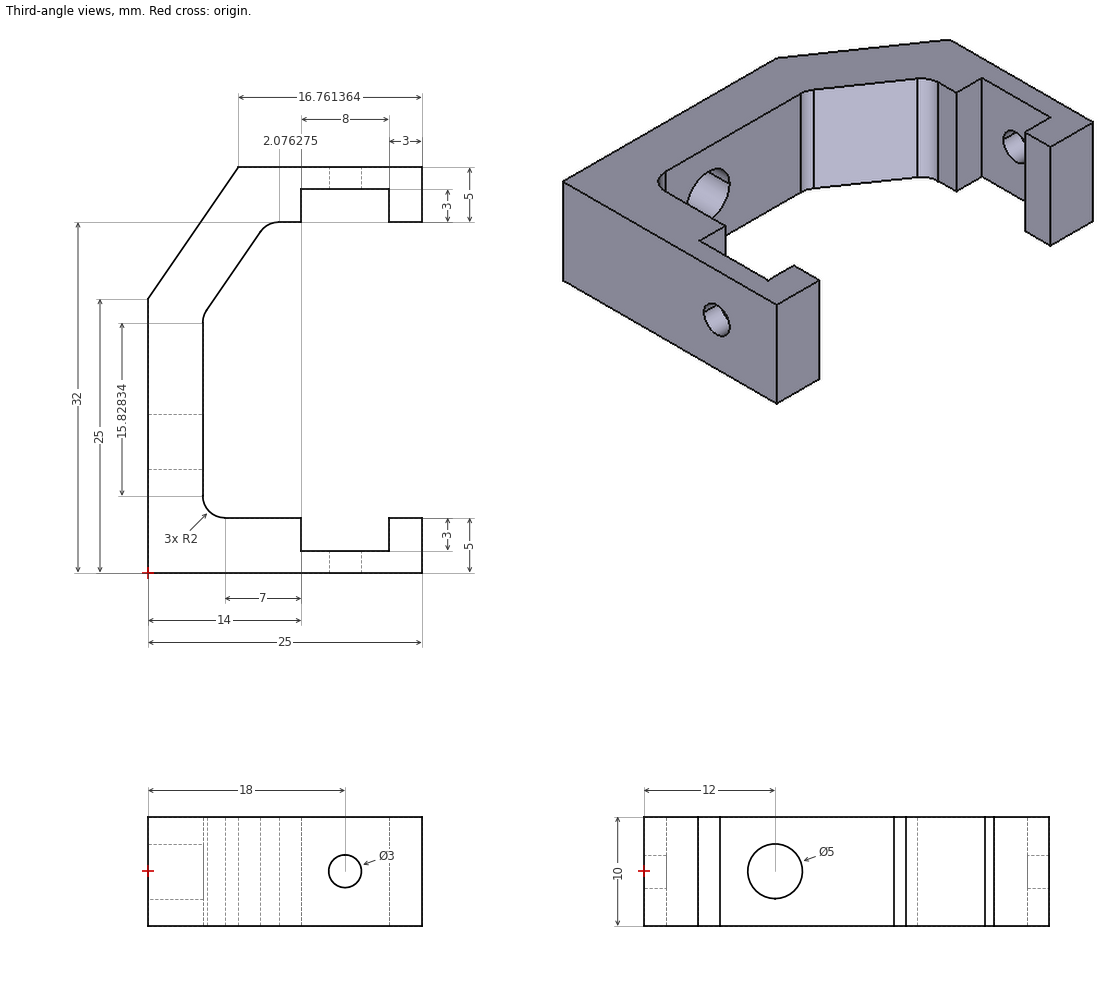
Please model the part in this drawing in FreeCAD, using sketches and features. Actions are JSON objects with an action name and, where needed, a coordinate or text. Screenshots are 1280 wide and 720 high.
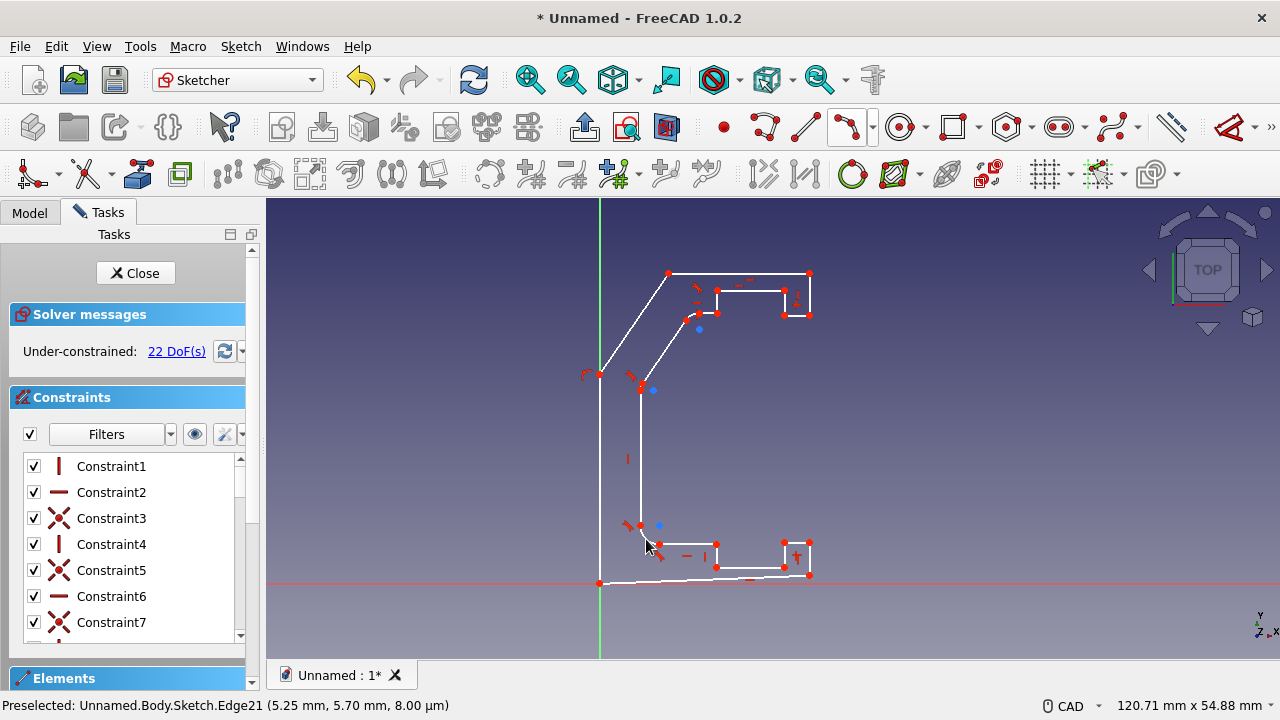
{"action": "left_click", "coordinate": [663, 581]}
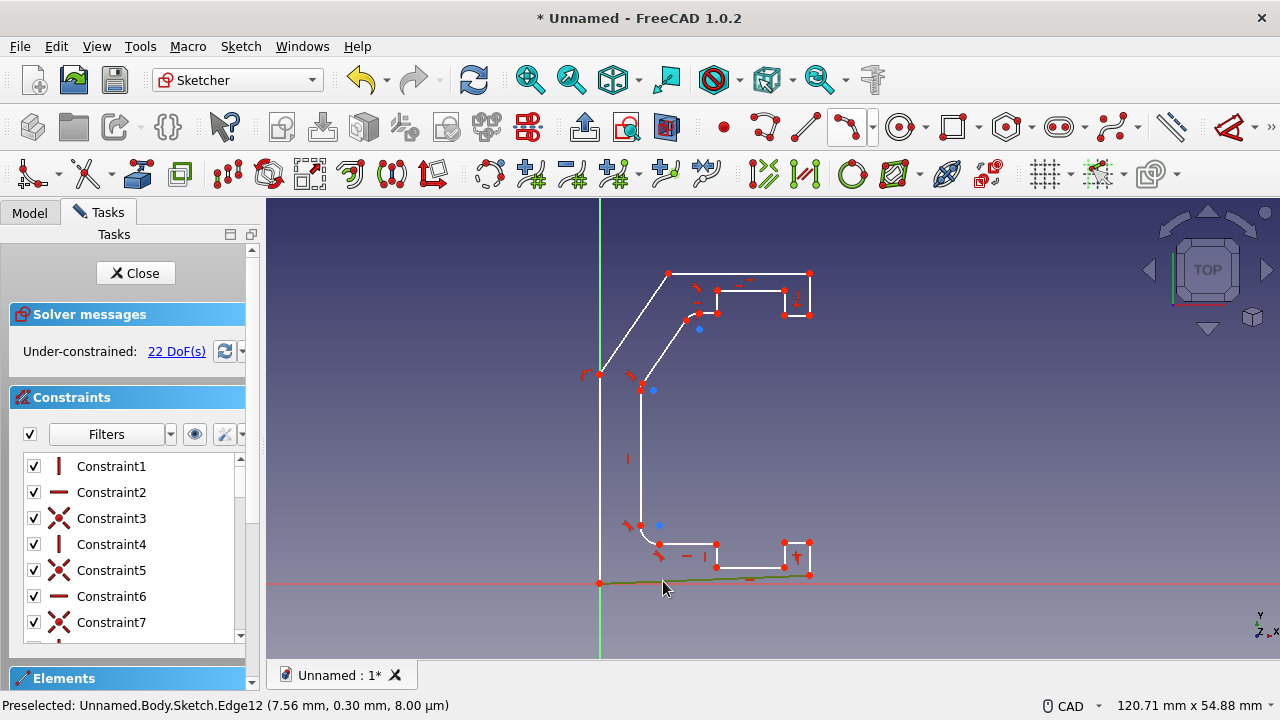
{"action": "key", "text": "h"}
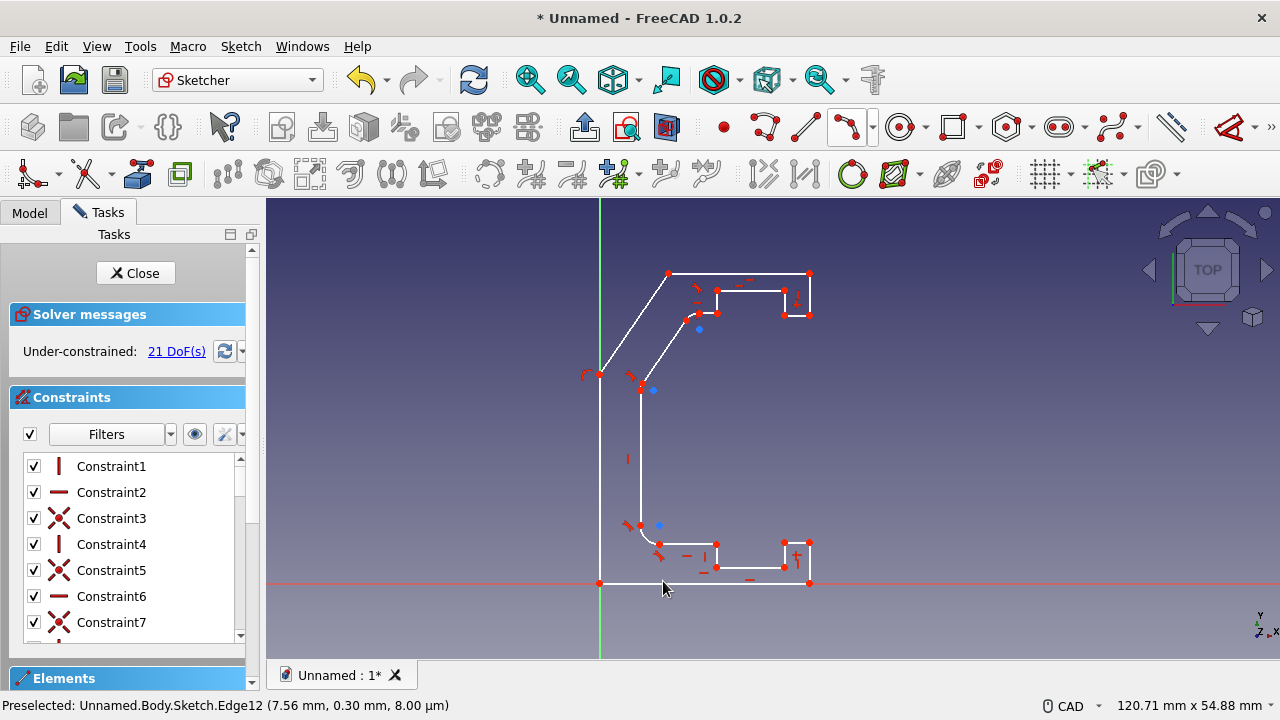
{"action": "scroll", "coordinate": [641, 387], "scroll_direction": "up", "scroll_amount": 7}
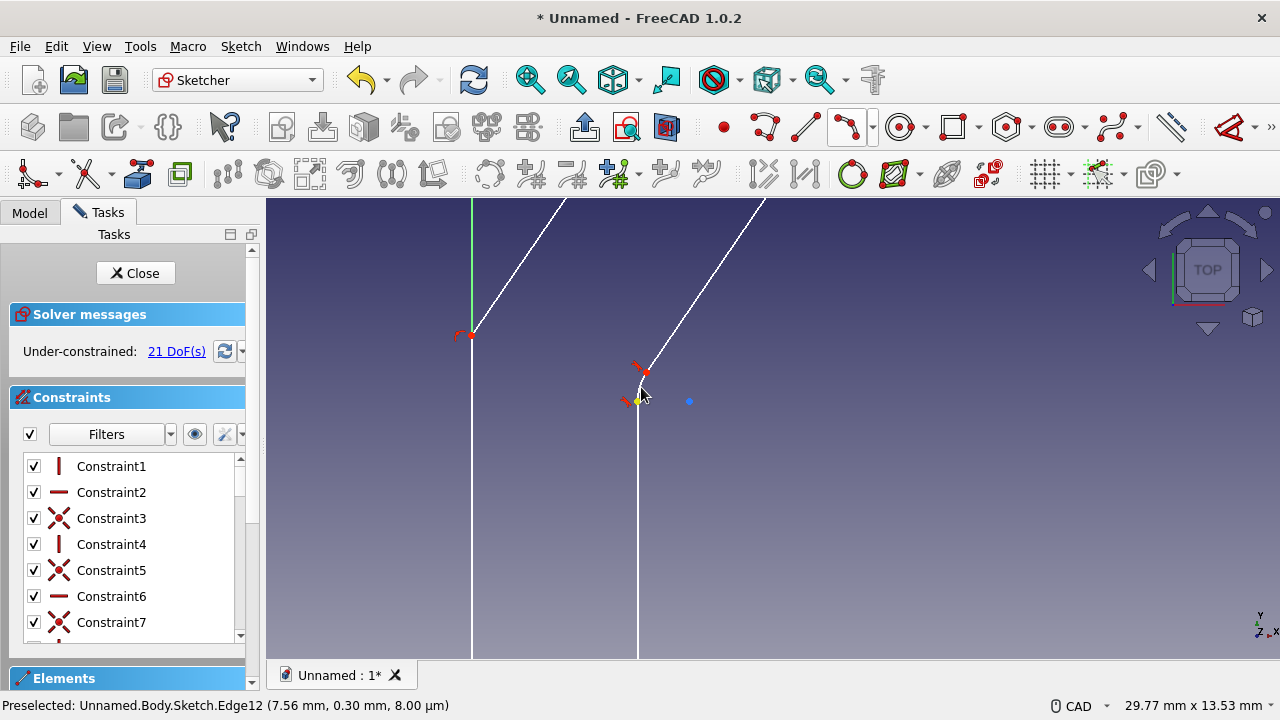
{"action": "left_click", "coordinate": [640, 386]}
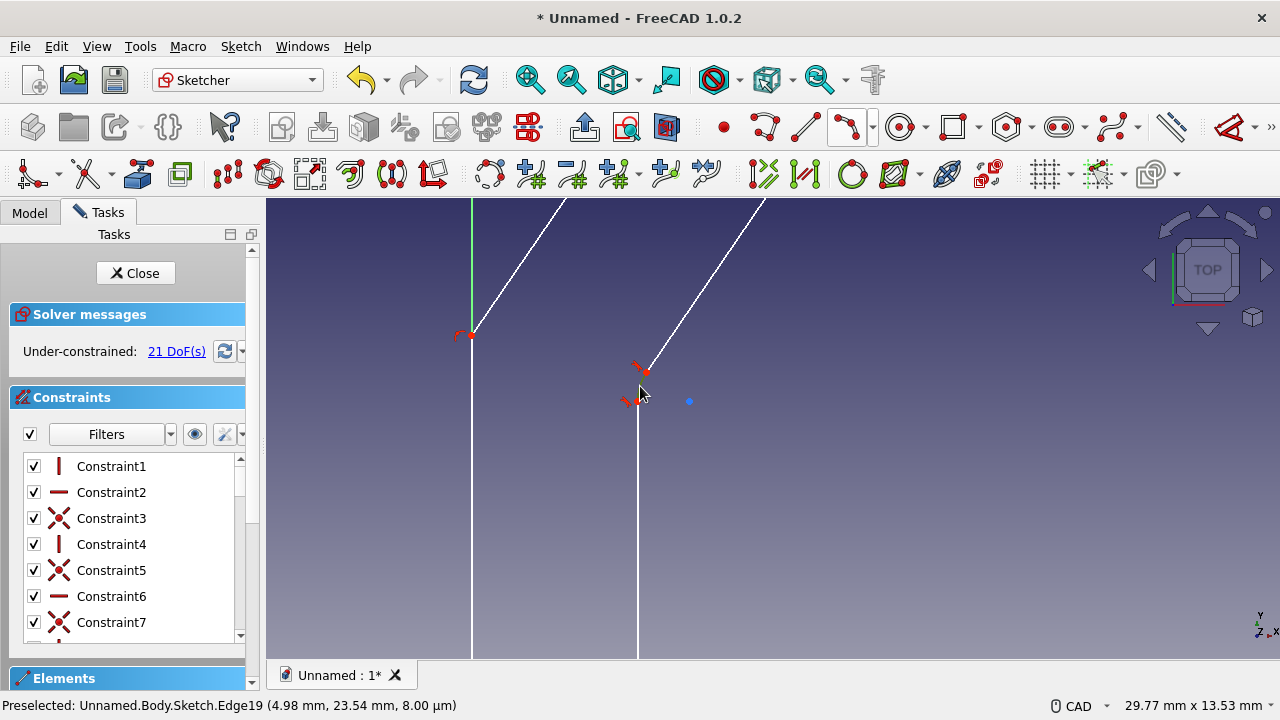
{"action": "scroll", "coordinate": [641, 387], "scroll_direction": "down", "scroll_amount": 7}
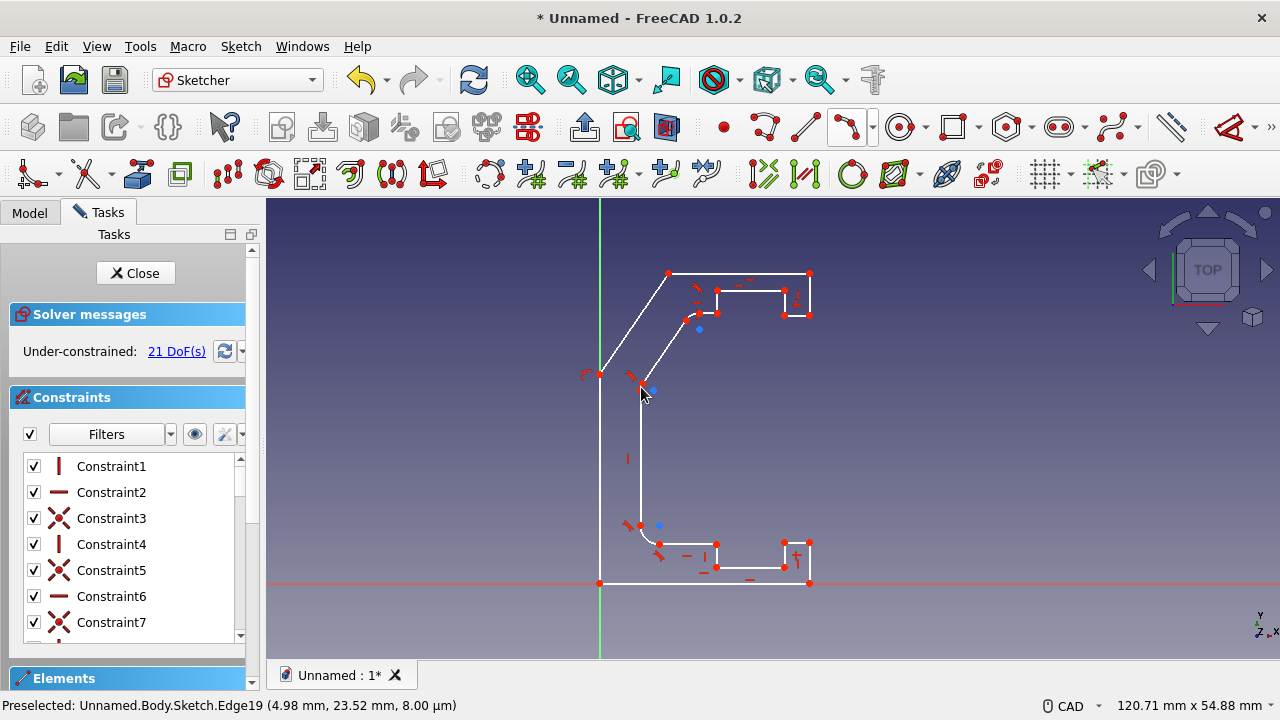
{"action": "scroll", "coordinate": [695, 314], "scroll_direction": "up", "scroll_amount": 6}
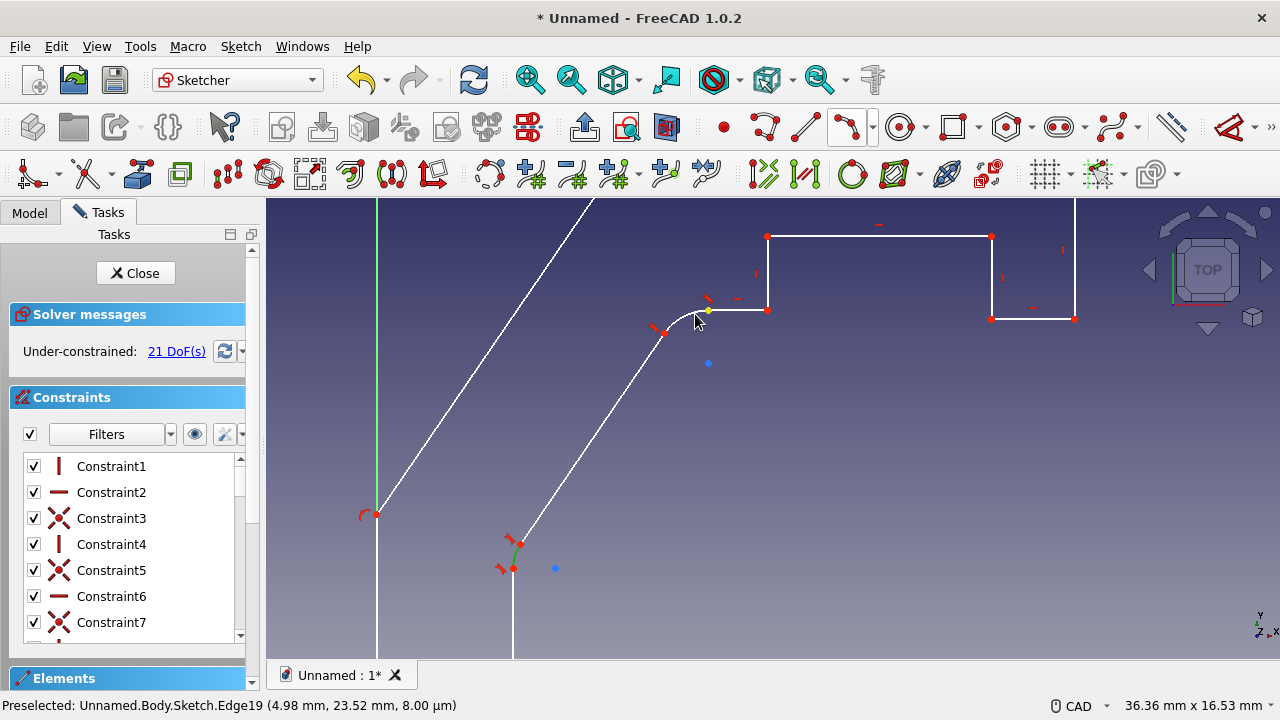
{"action": "left_click", "coordinate": [693, 313]}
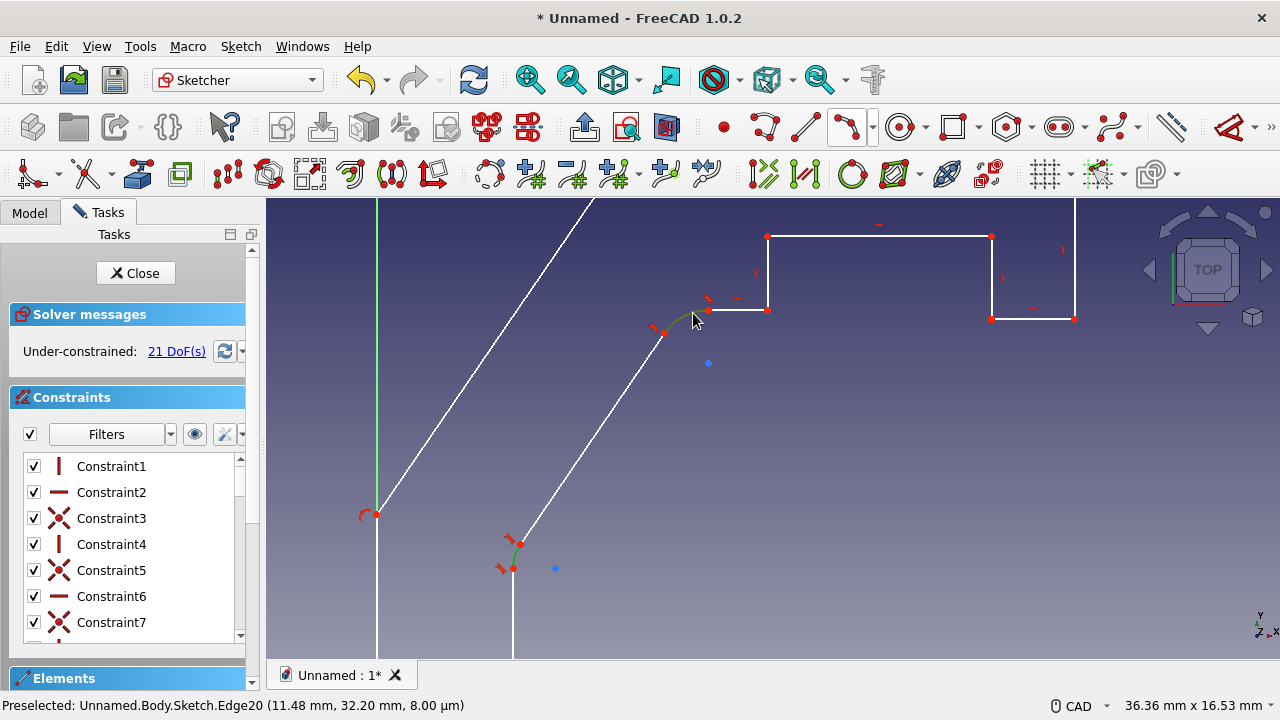
{"action": "scroll", "coordinate": [695, 314], "scroll_direction": "down", "scroll_amount": 6}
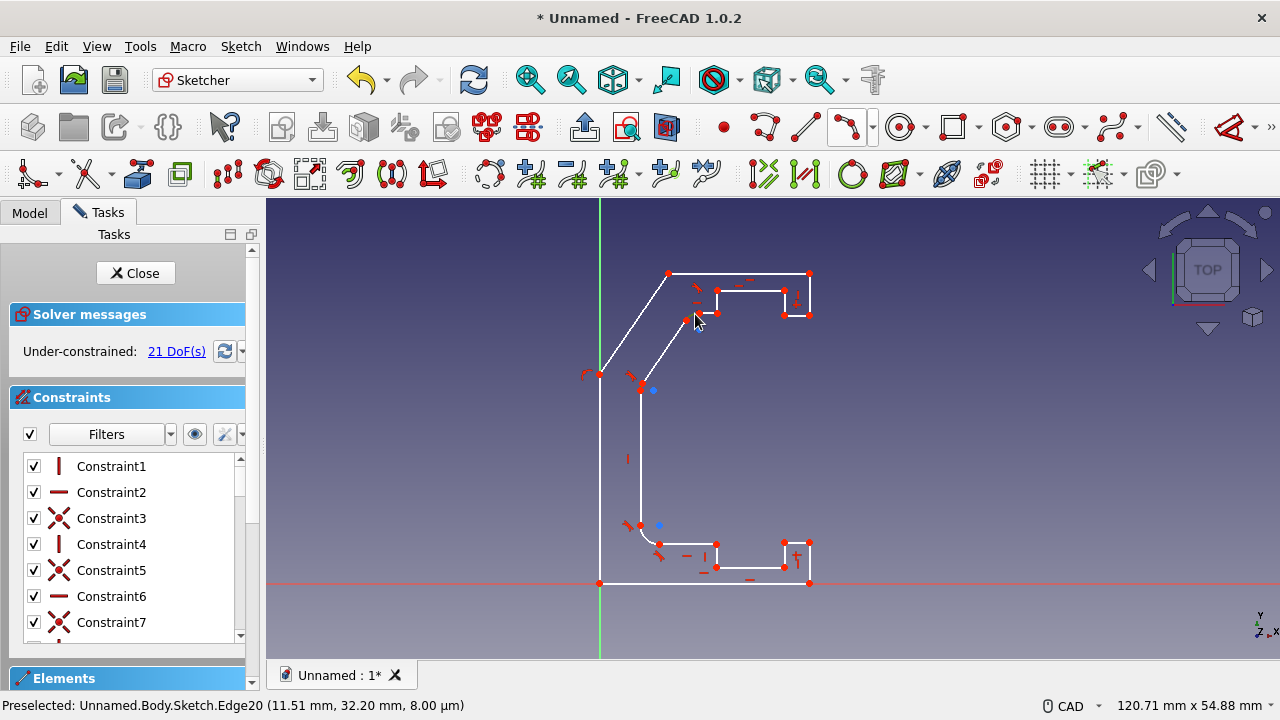
{"action": "scroll", "coordinate": [643, 534], "scroll_direction": "up", "scroll_amount": 3}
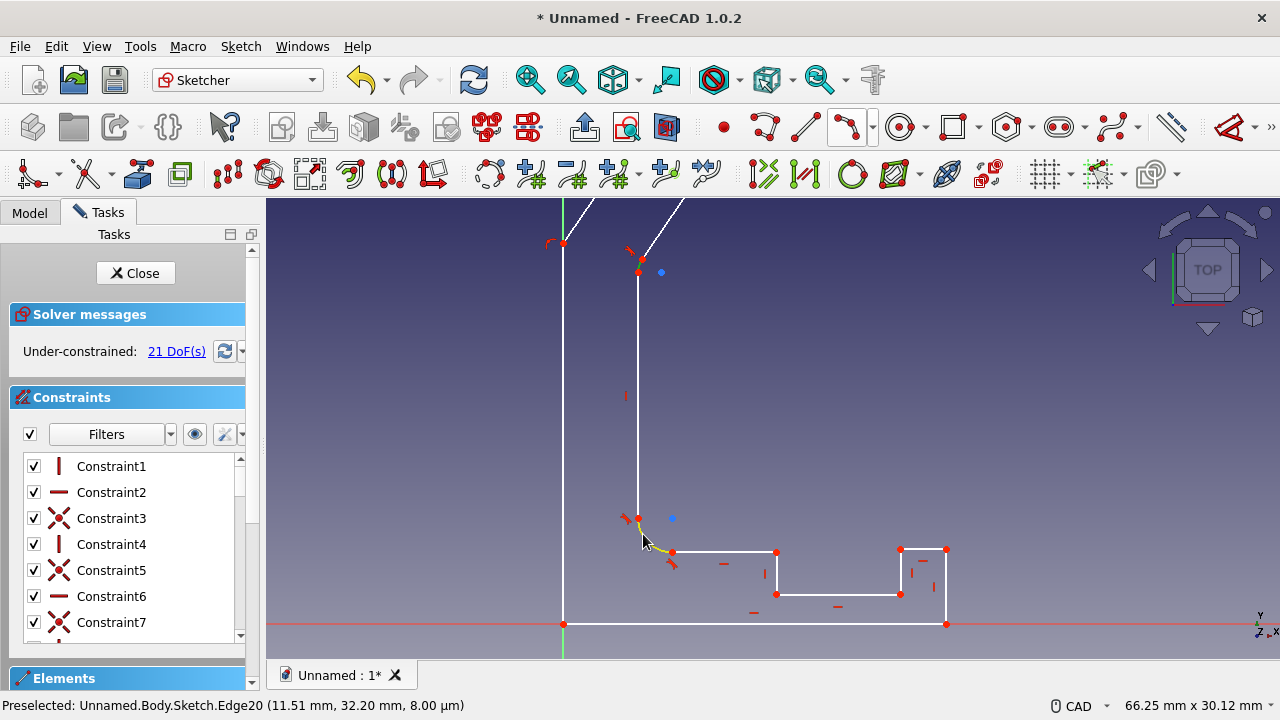
{"action": "left_click", "coordinate": [642, 534]}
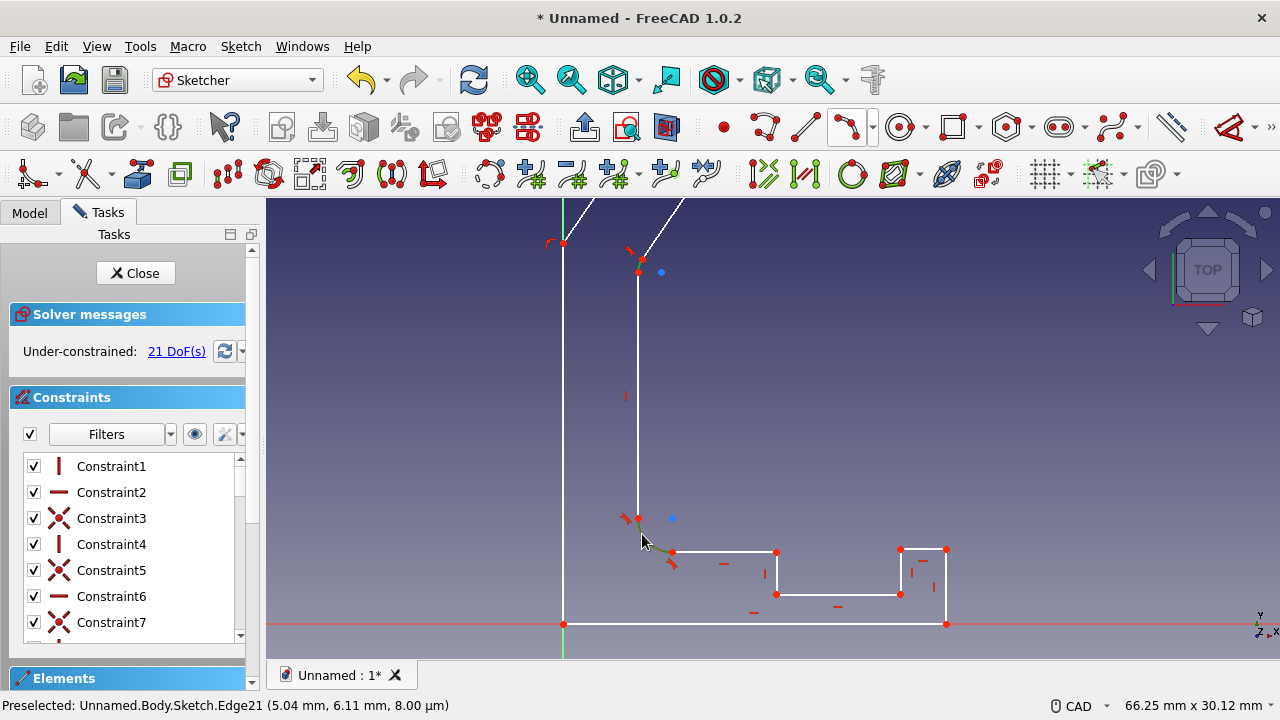
{"action": "key", "text": "e"}